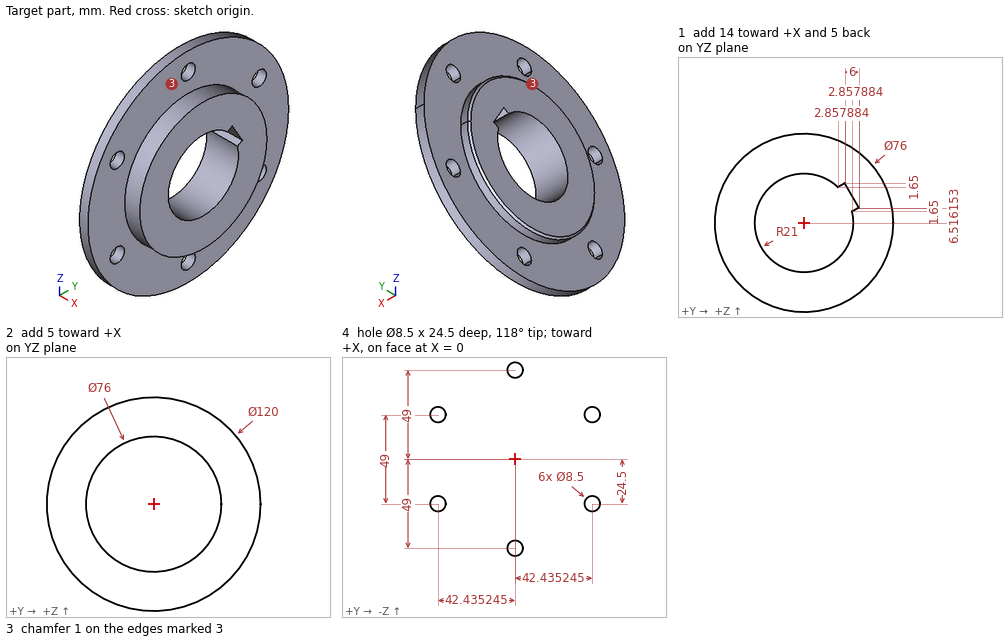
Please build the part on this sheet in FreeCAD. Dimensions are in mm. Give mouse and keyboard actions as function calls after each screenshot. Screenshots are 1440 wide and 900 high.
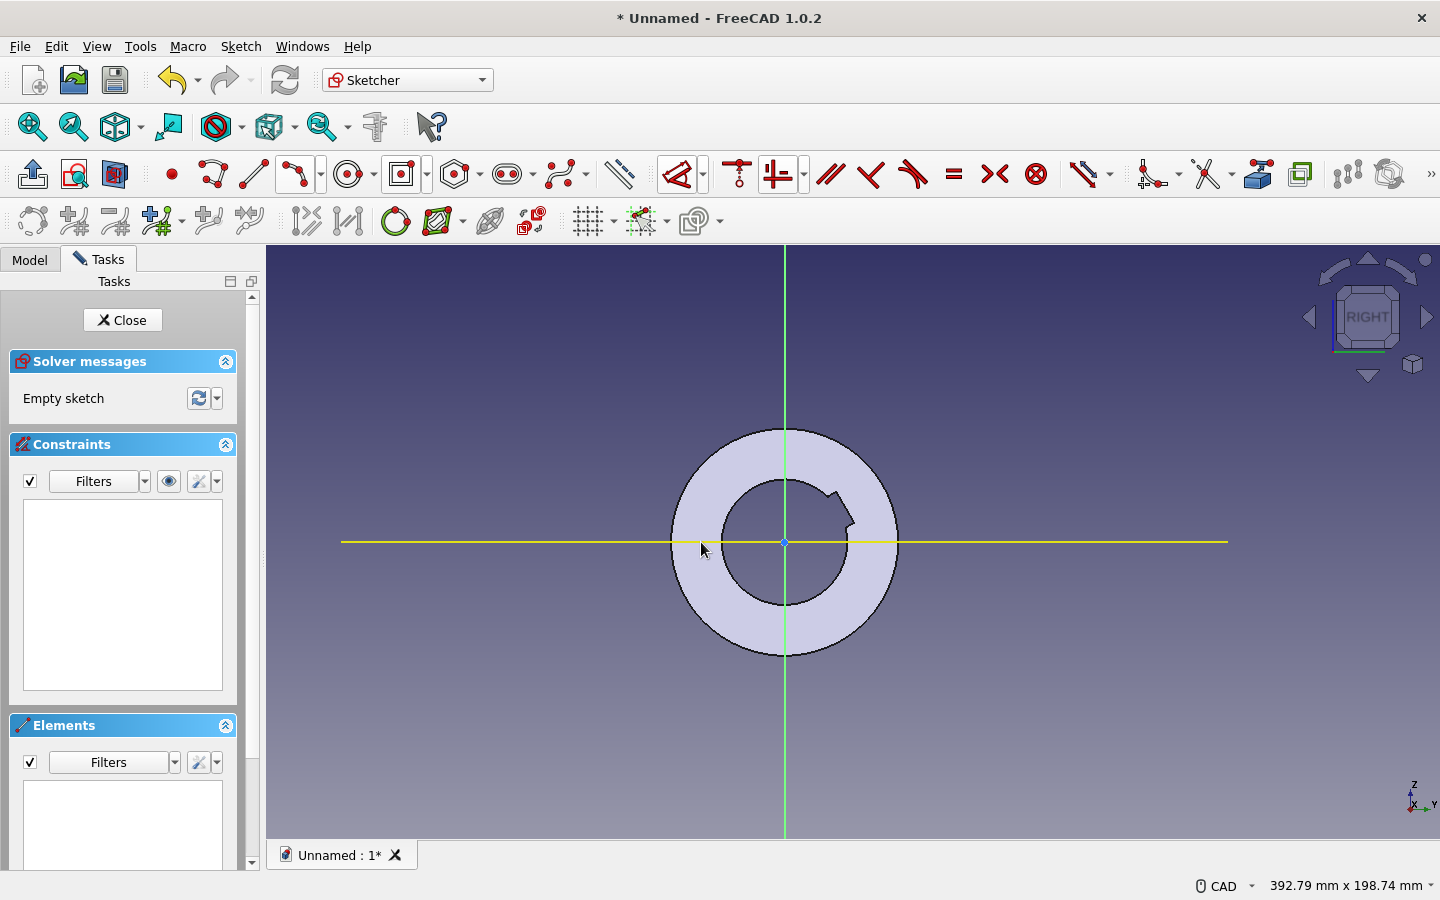
click(348, 174)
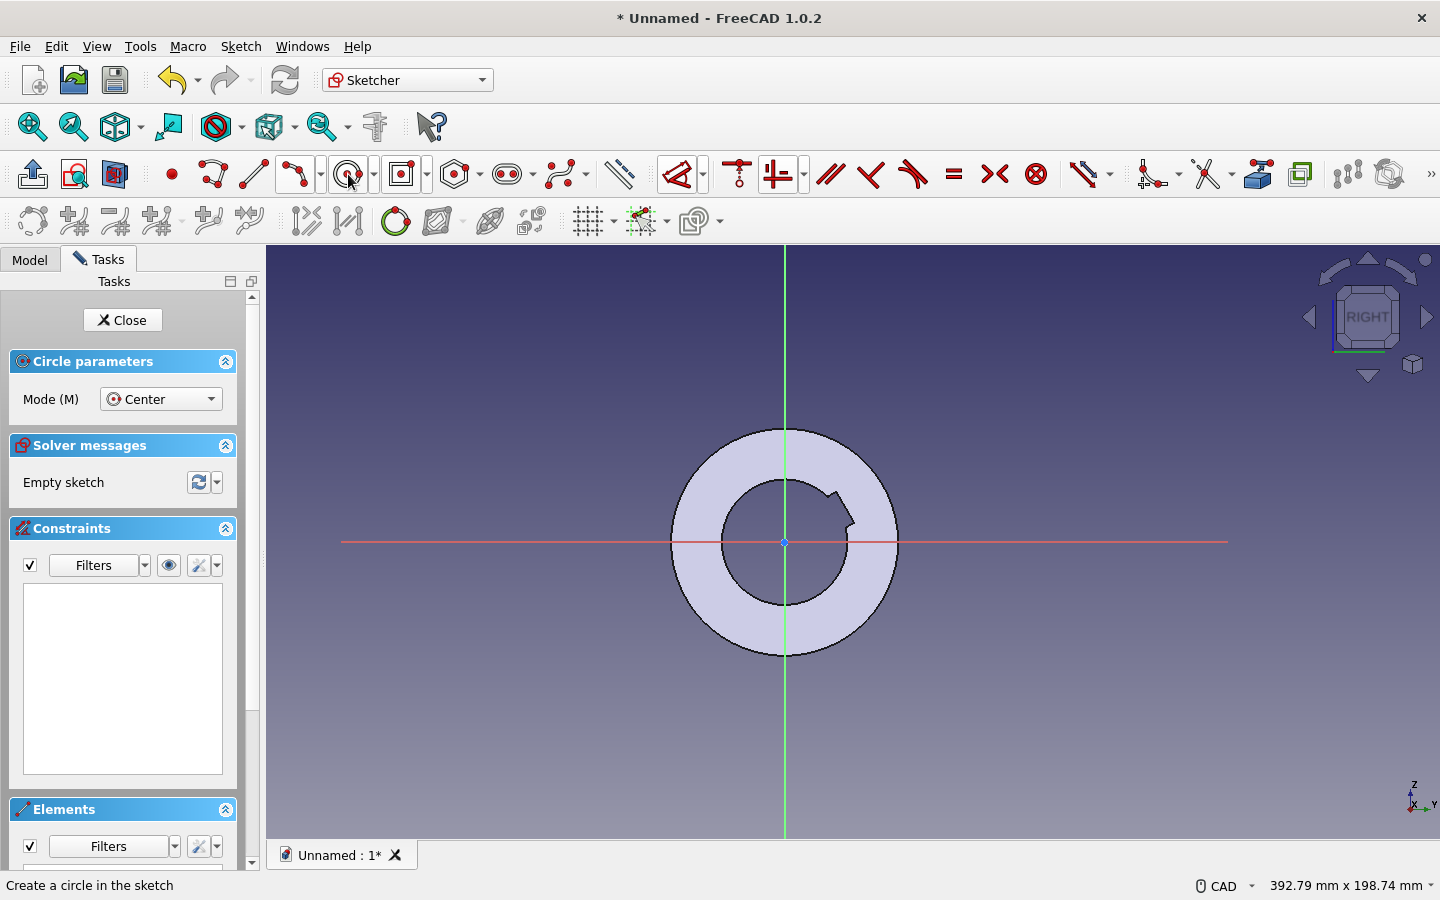
click(785, 542)
move(911, 415)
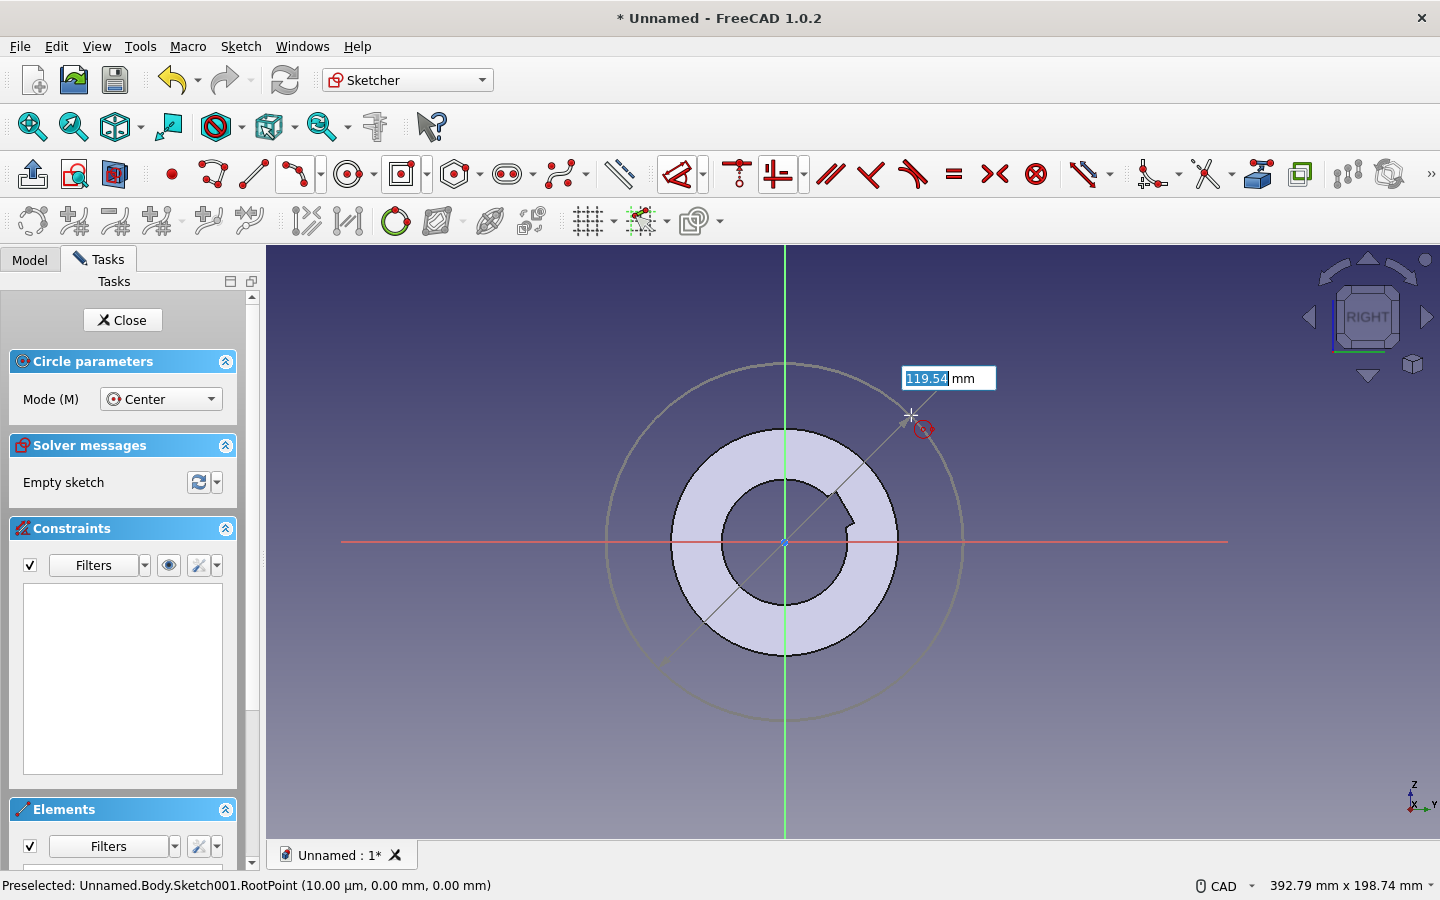
text(120)
key(Return)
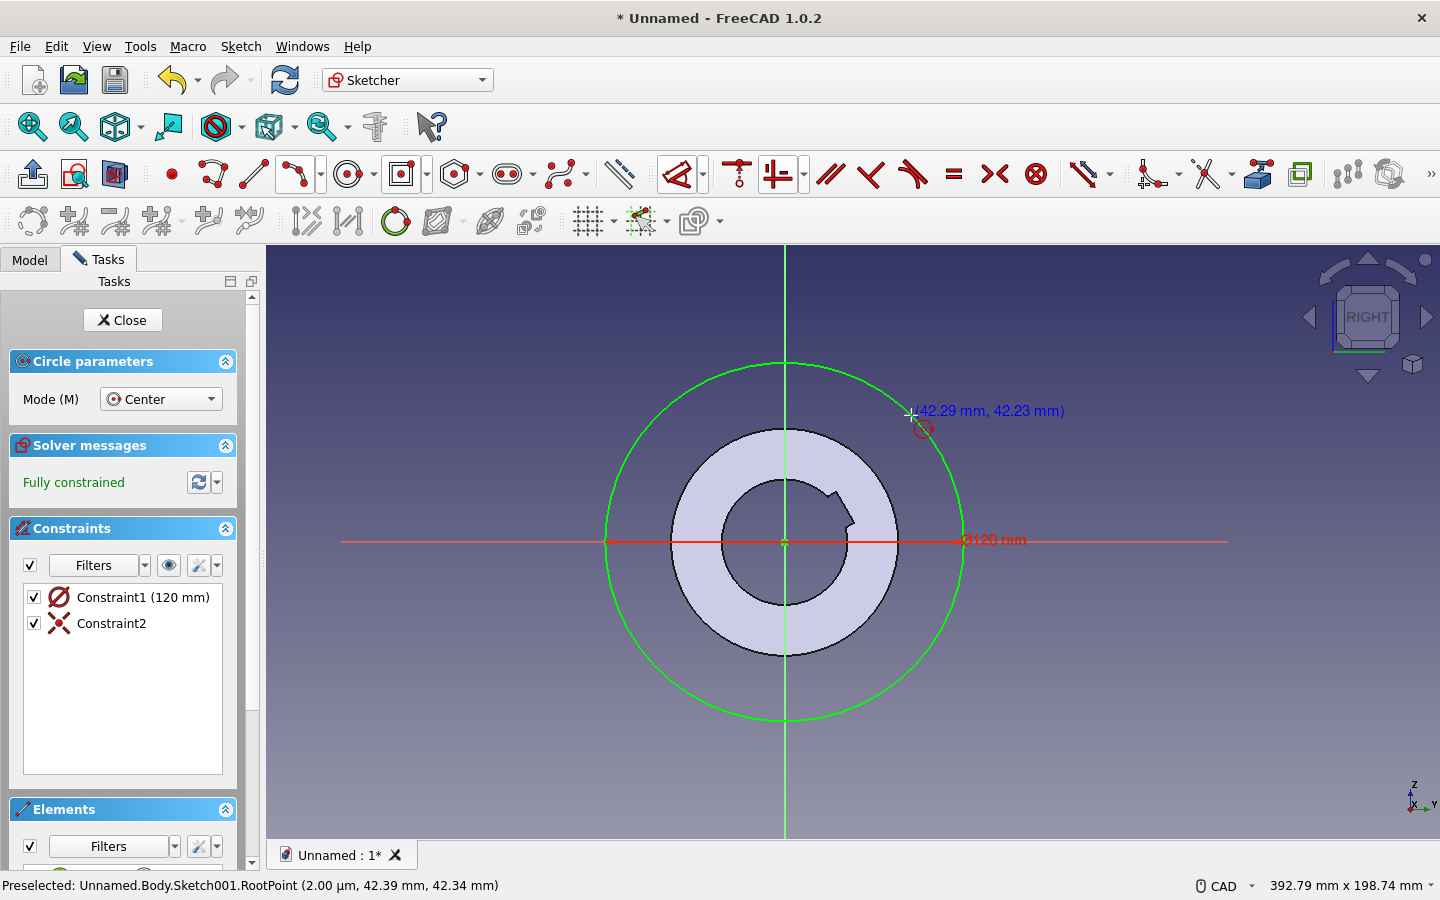
click(785, 542)
move(865, 462)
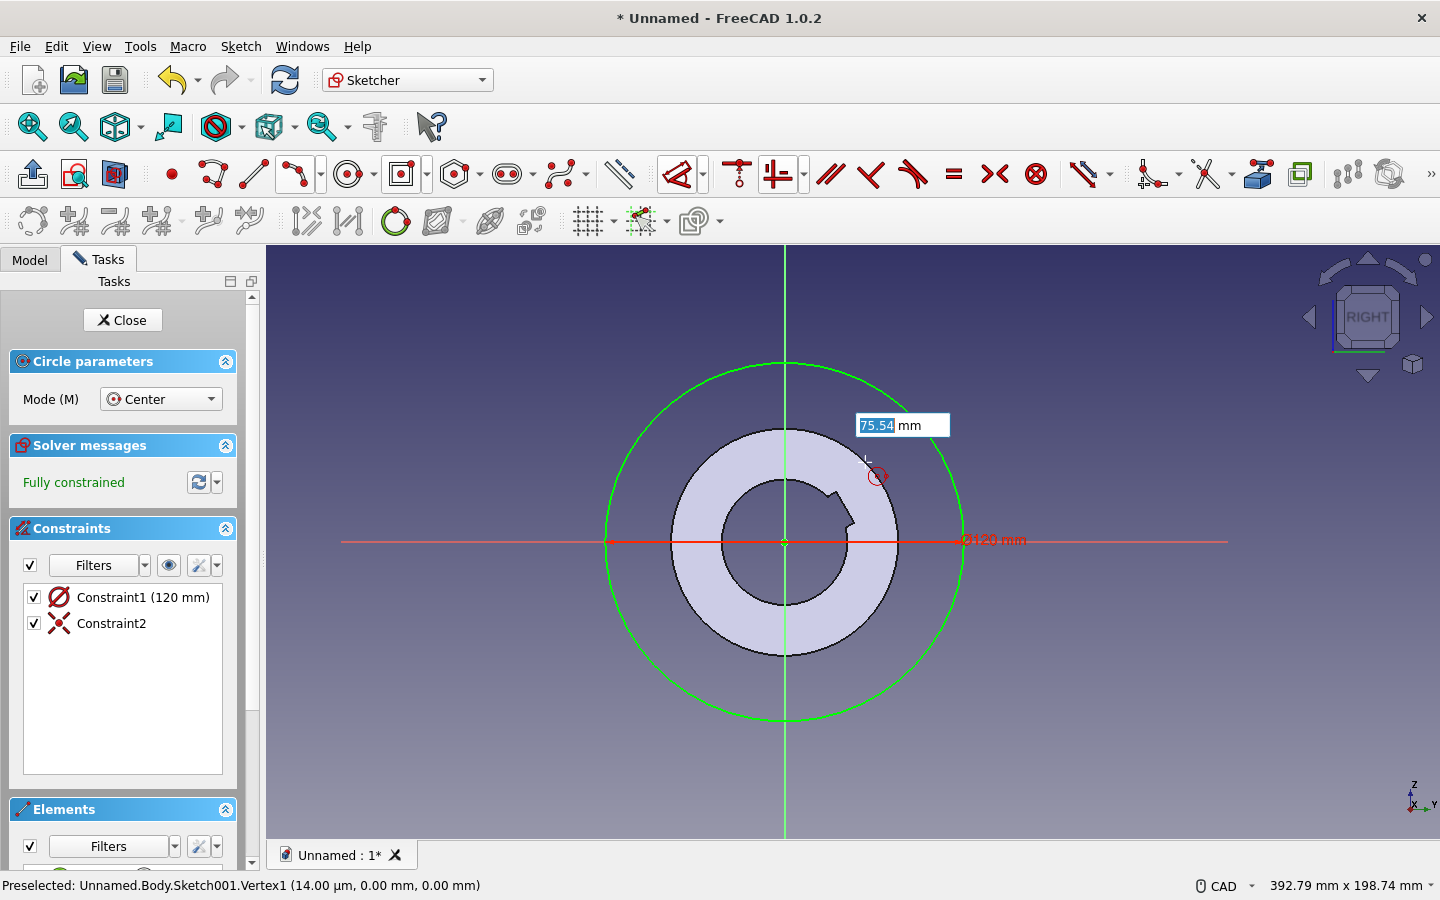
text(76)
key(Return)
key(Escape)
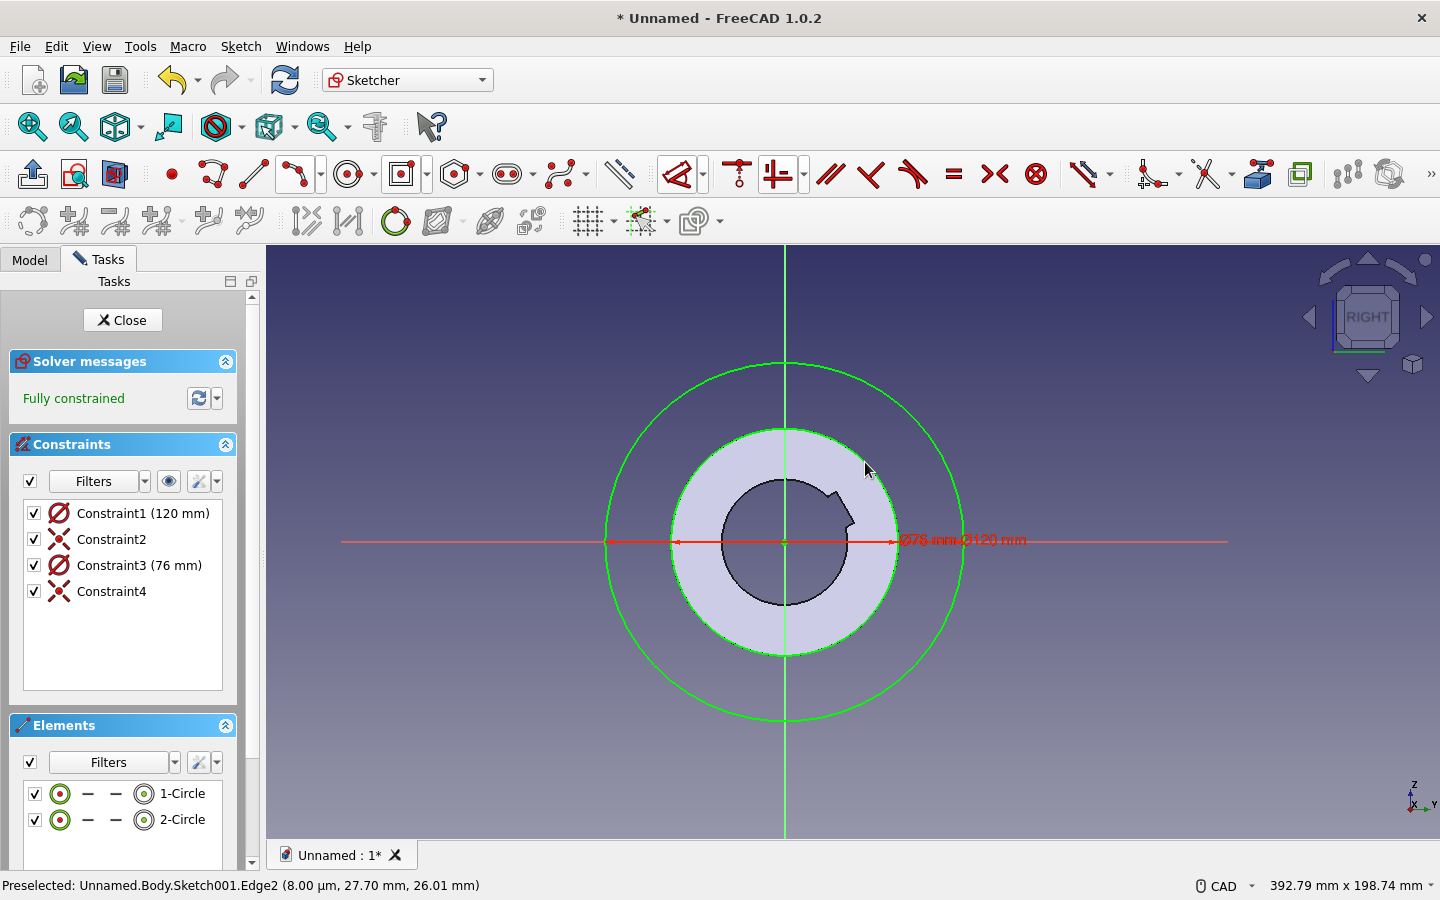
click(123, 320)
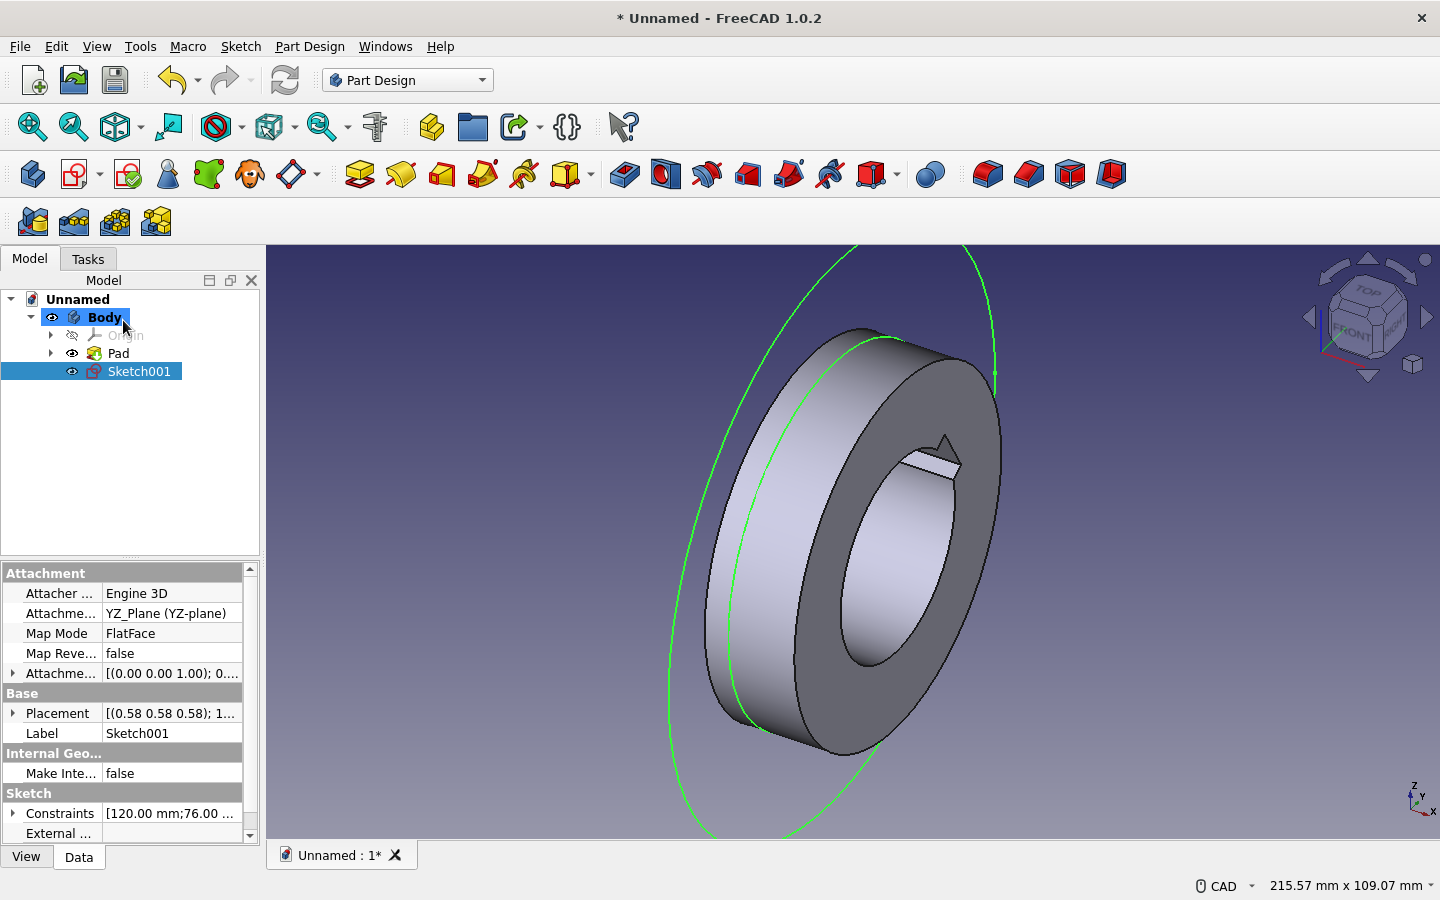
click(360, 174)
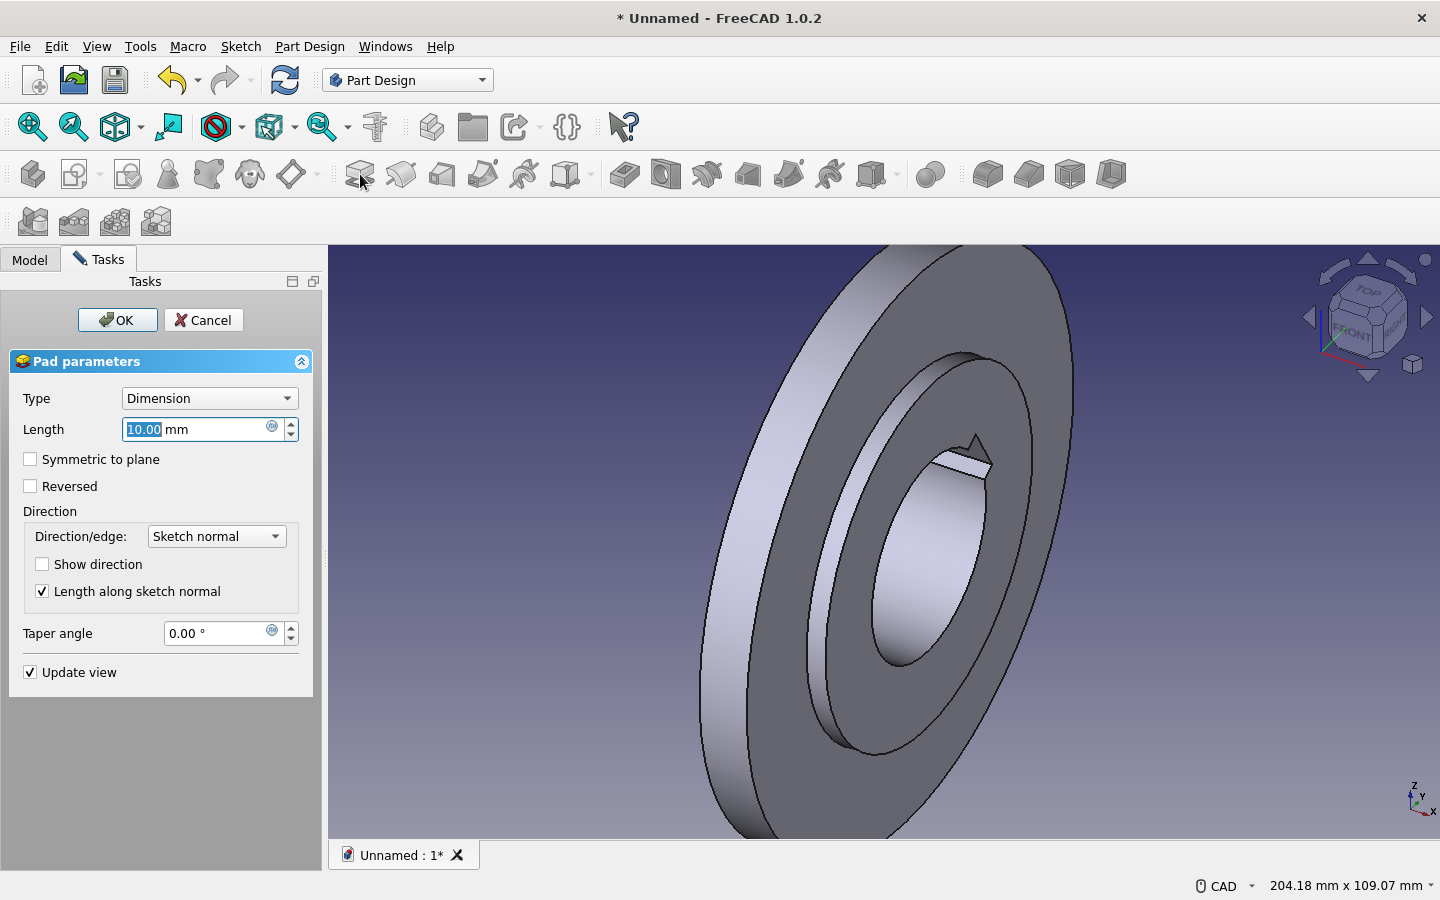
text(5)
key(Tab)